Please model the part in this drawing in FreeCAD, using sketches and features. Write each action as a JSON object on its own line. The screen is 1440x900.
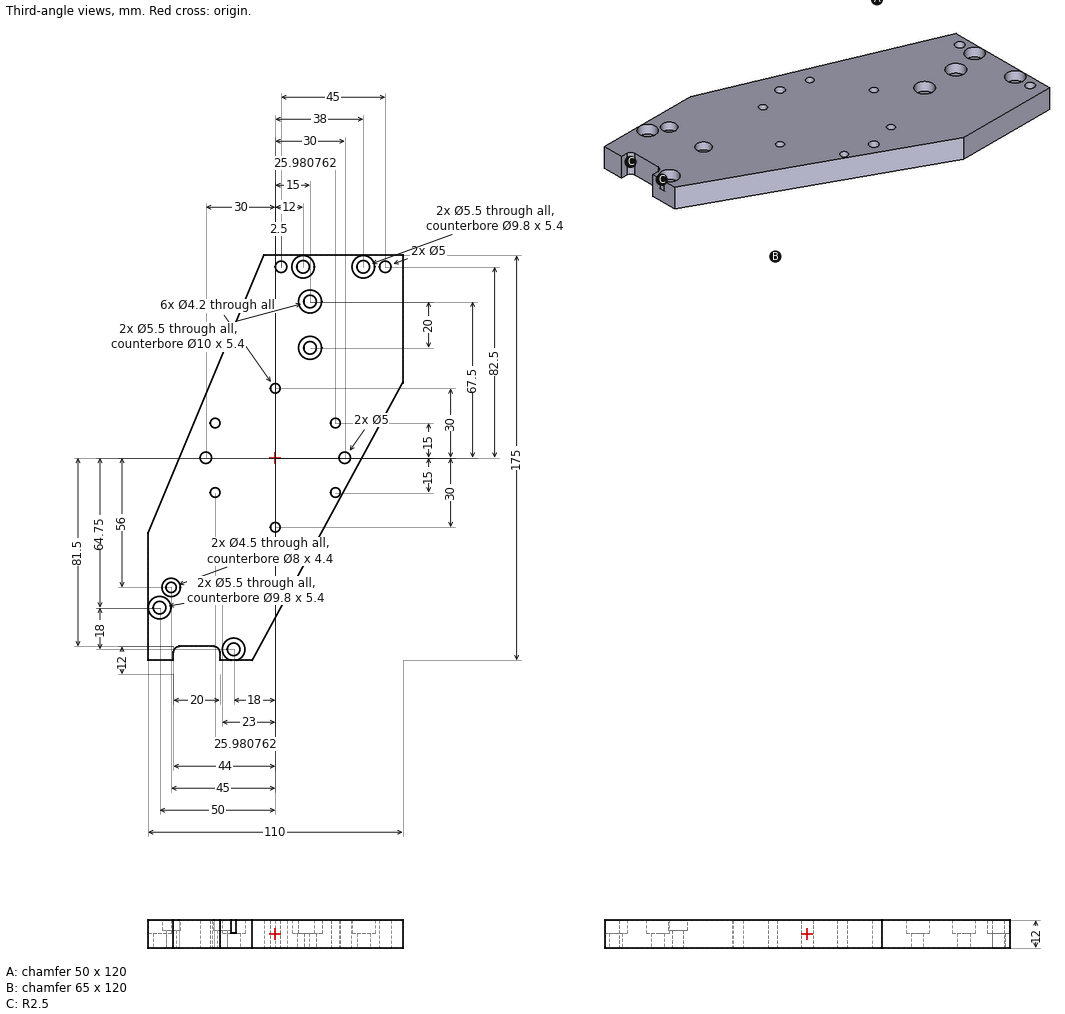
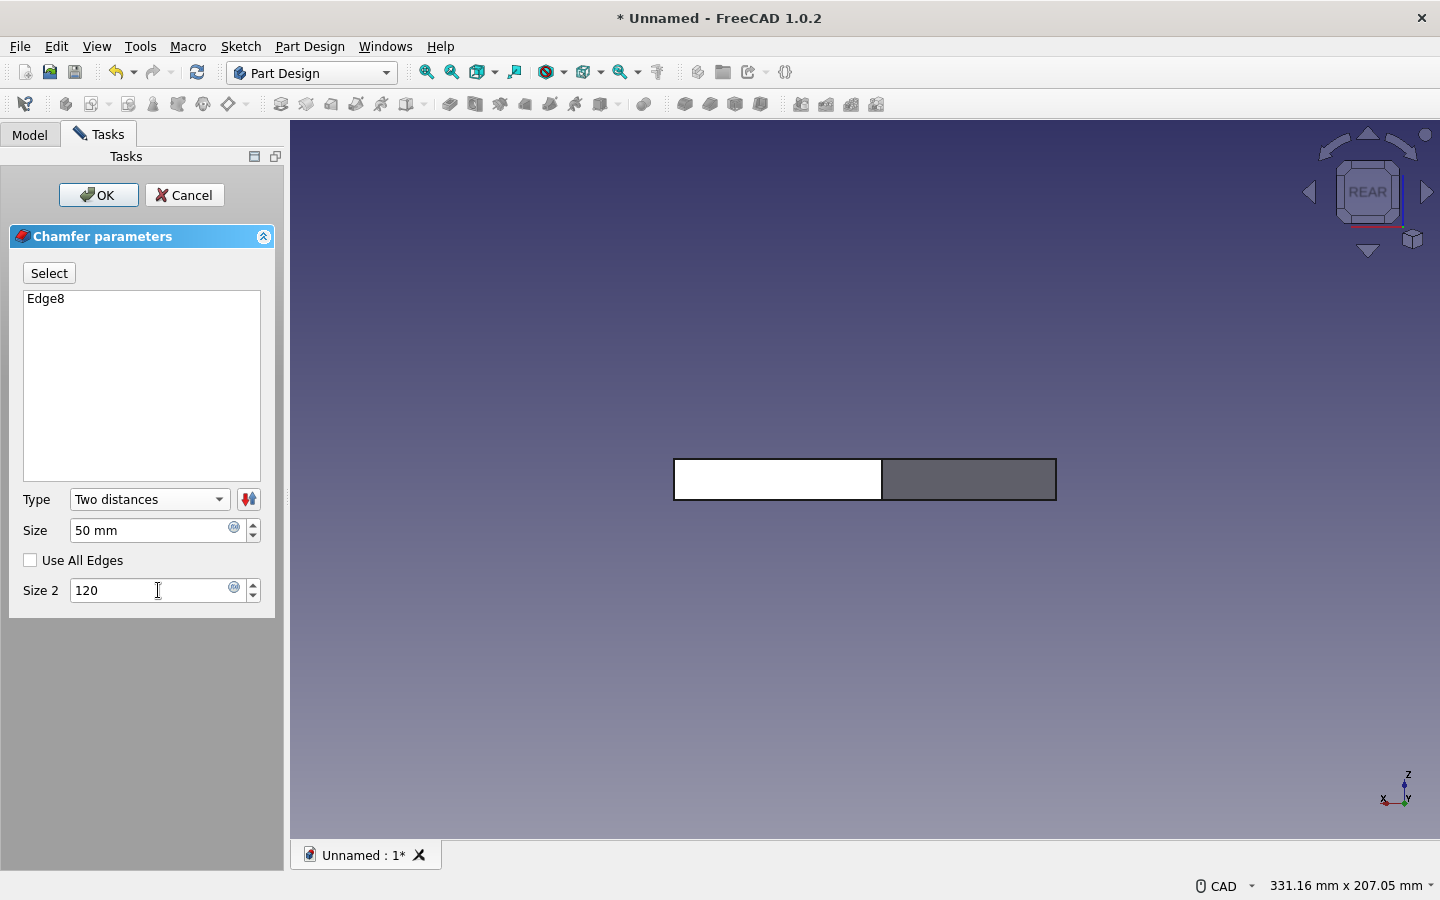
{"action": "left_click", "coordinate": [99, 195]}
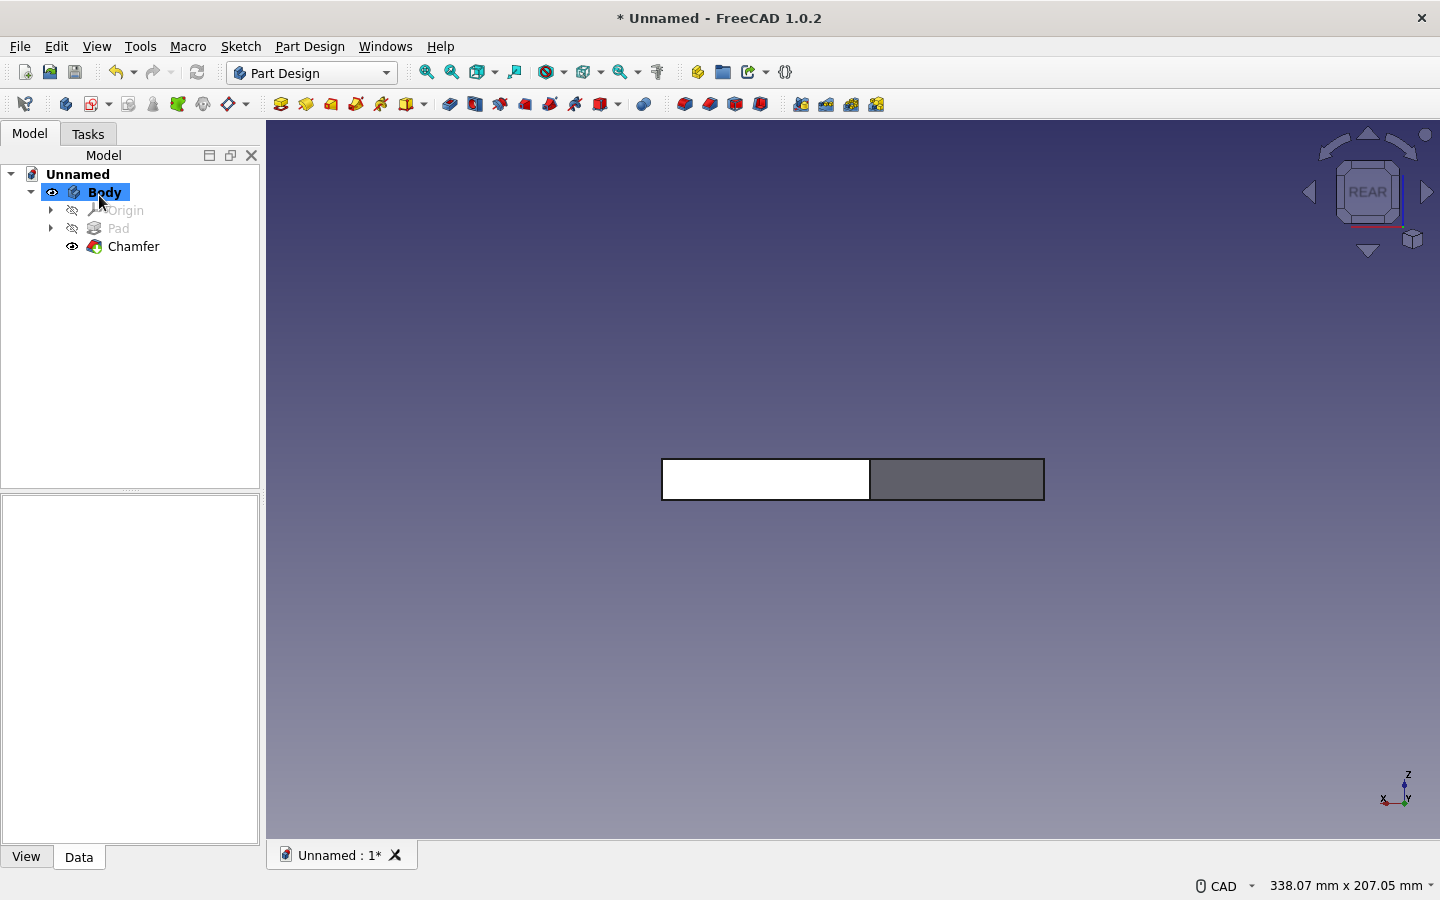
{"action": "left_click", "coordinate": [427, 72]}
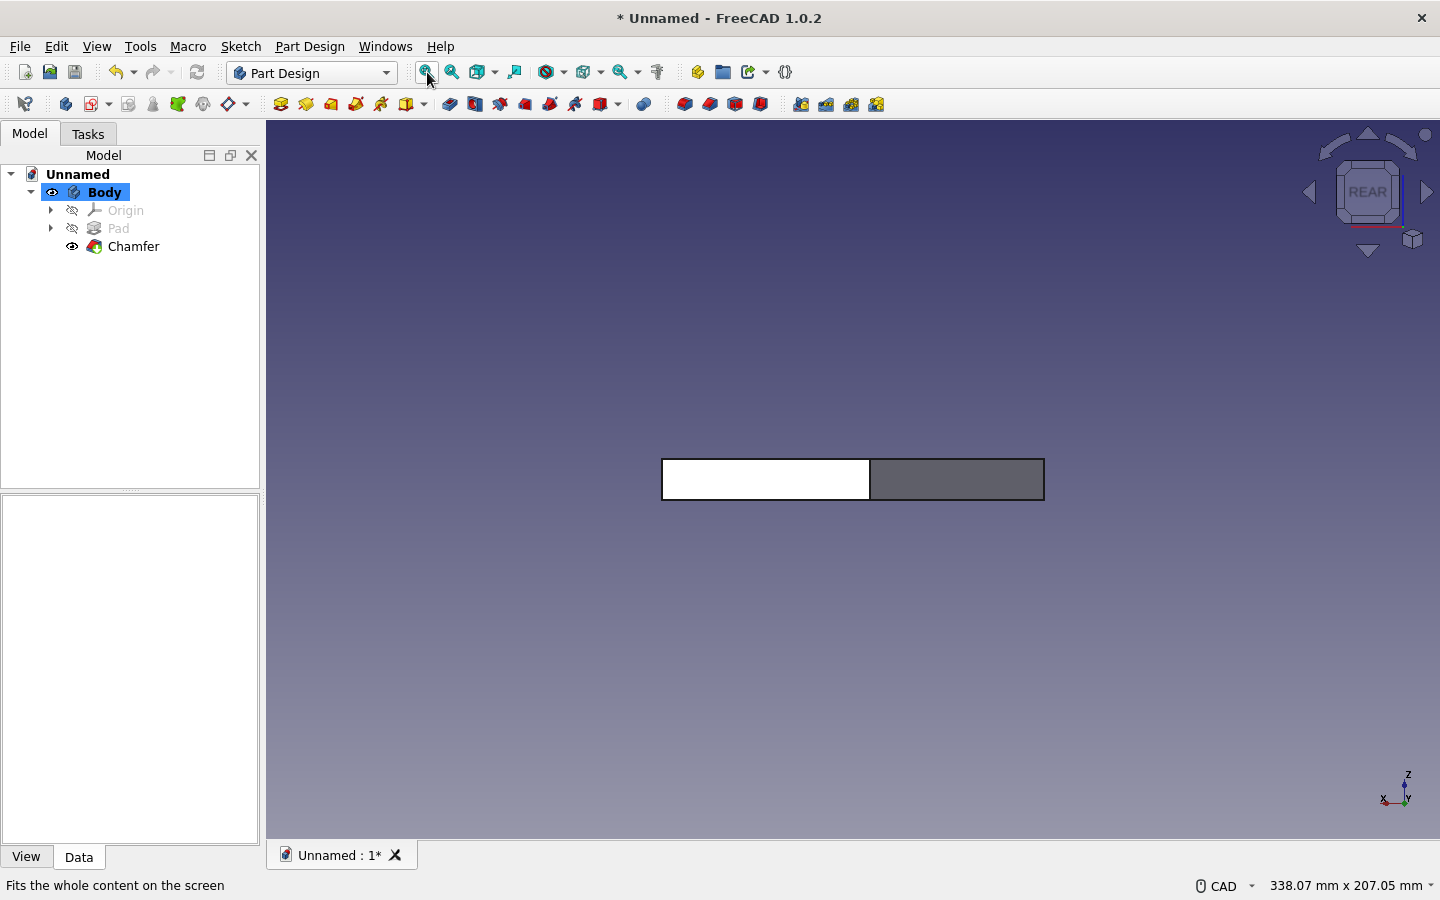
{"action": "key", "text": "0"}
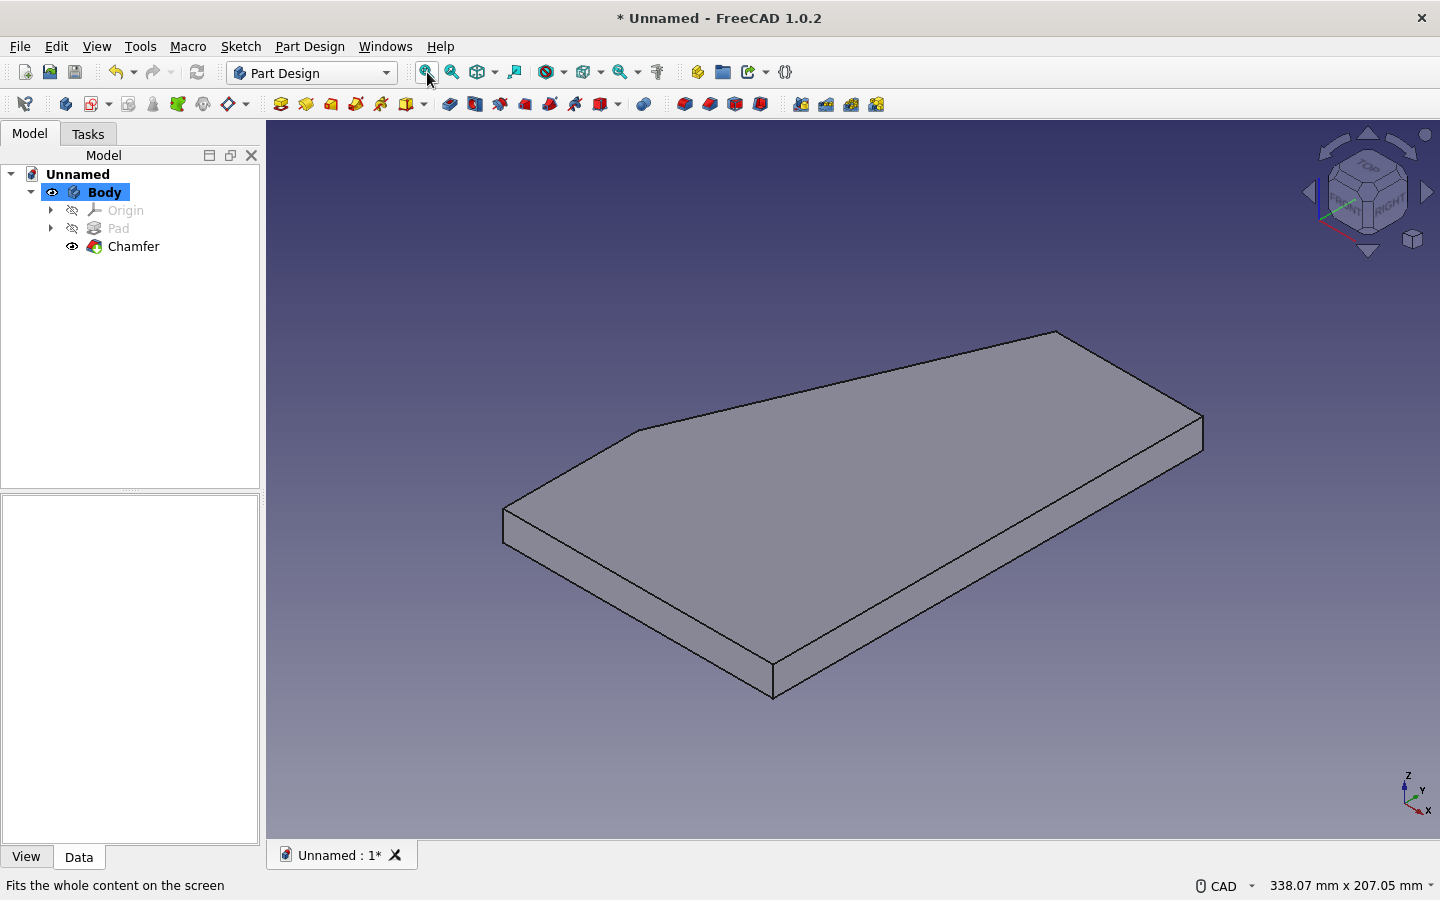
{"action": "left_click", "coordinate": [773, 681]}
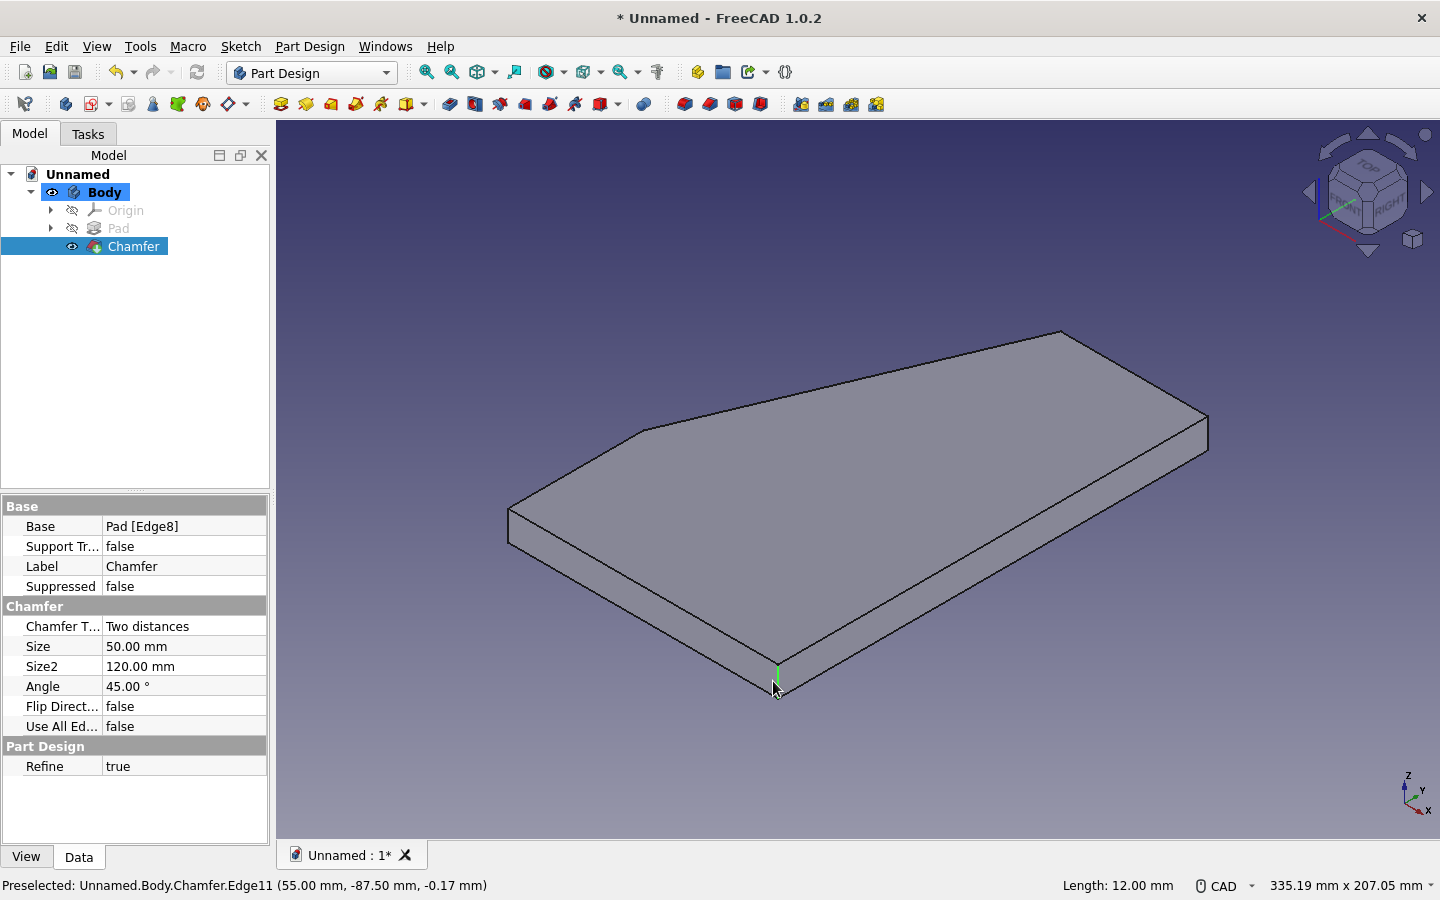
{"action": "left_click", "coordinate": [710, 104]}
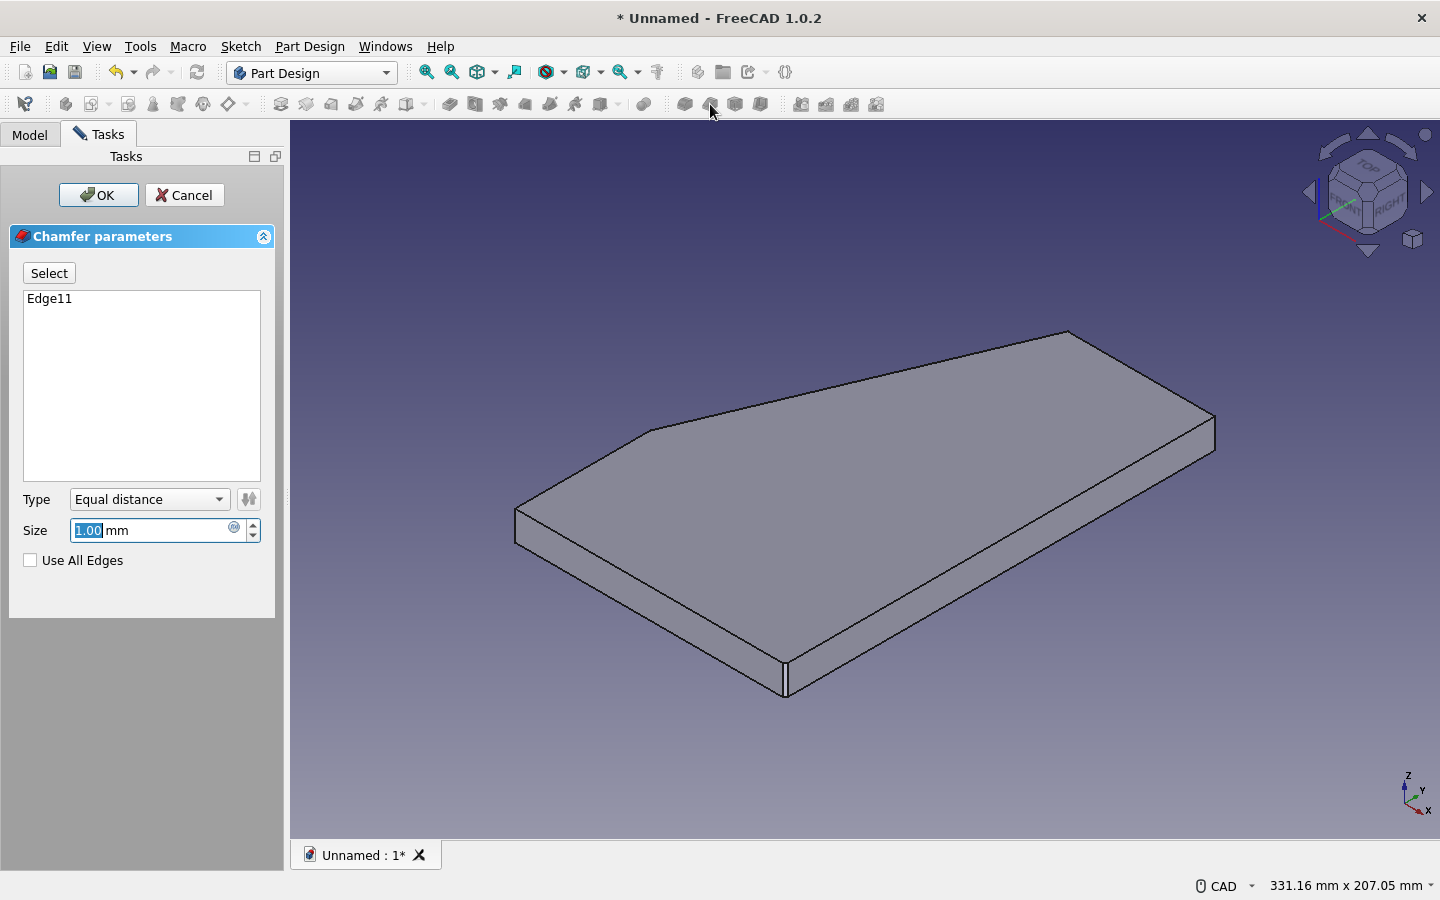
{"action": "type", "text": "65"}
{"action": "key", "text": "Tab"}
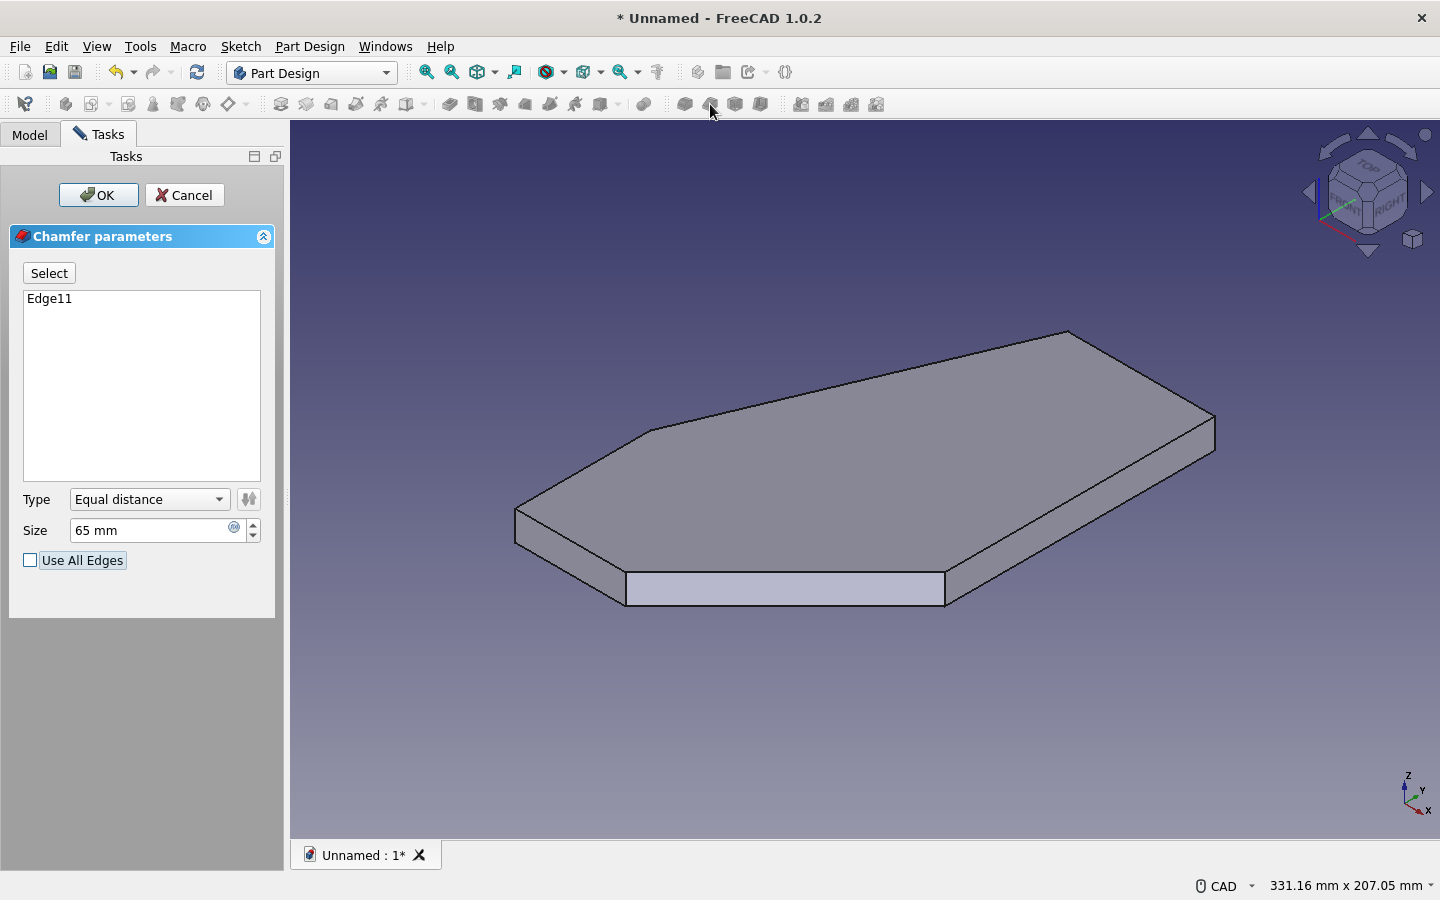
{"action": "left_click", "coordinate": [150, 500]}